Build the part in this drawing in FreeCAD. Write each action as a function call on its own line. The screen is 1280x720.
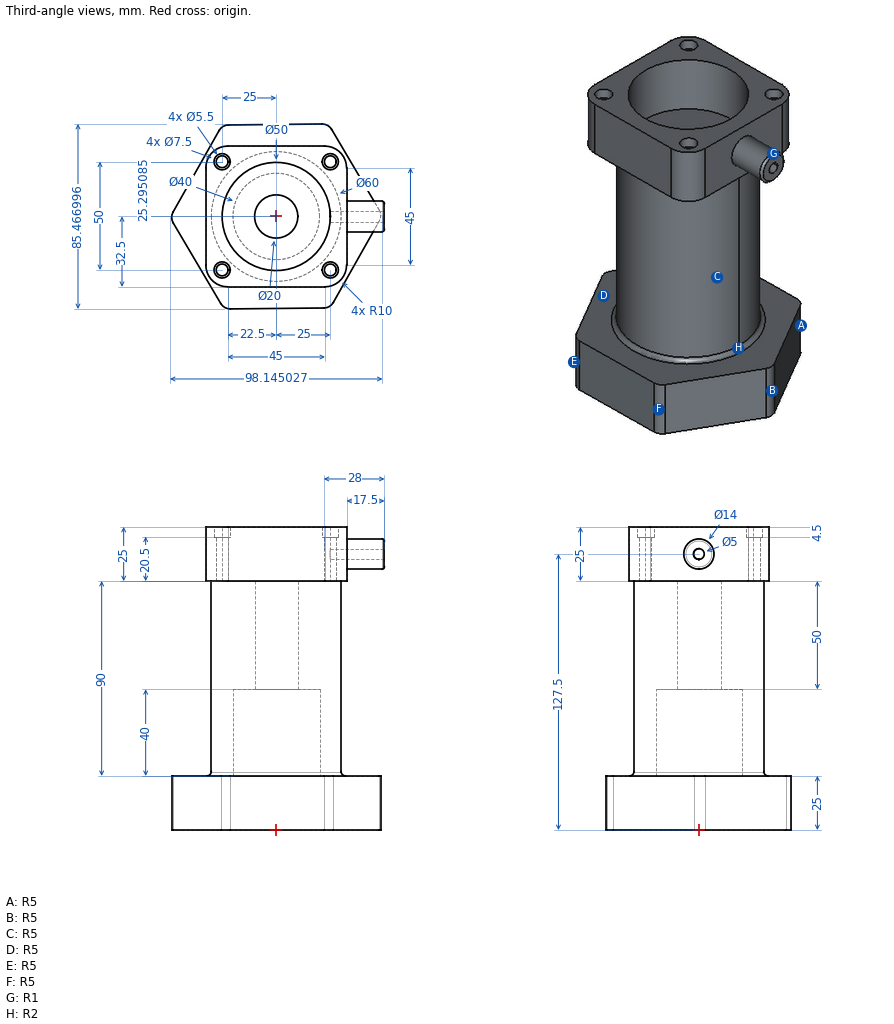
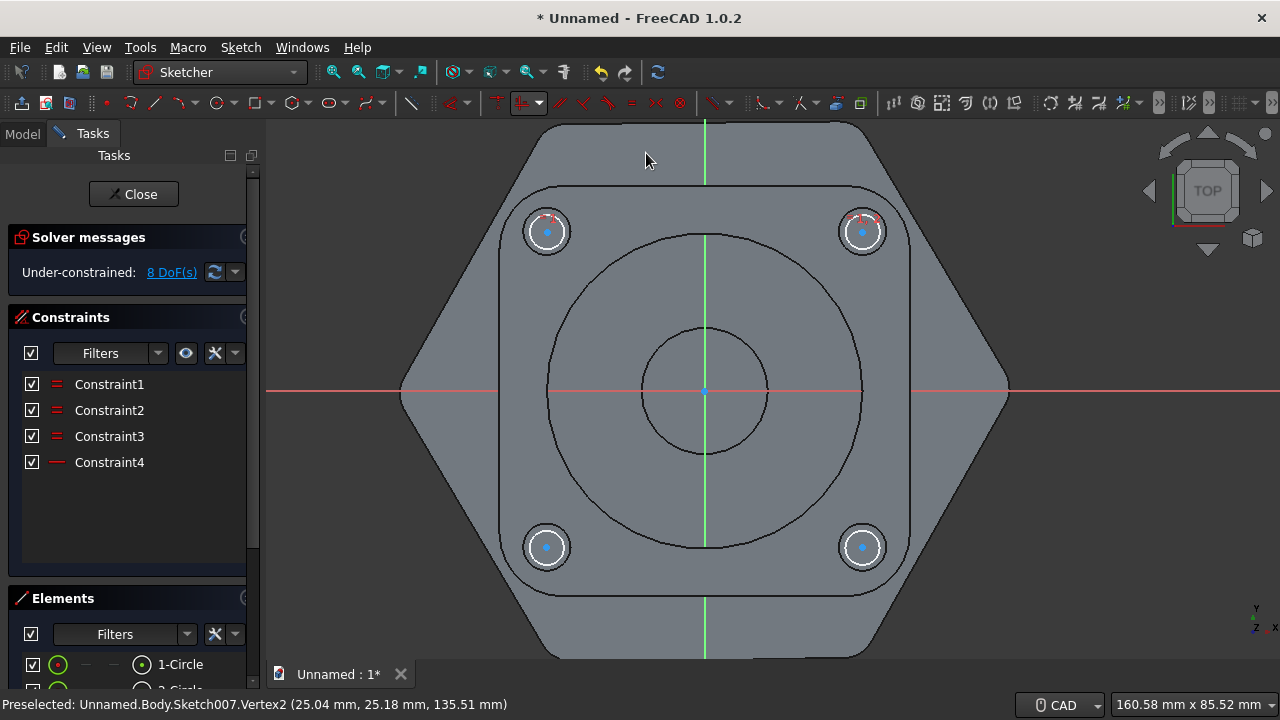
click(863, 232)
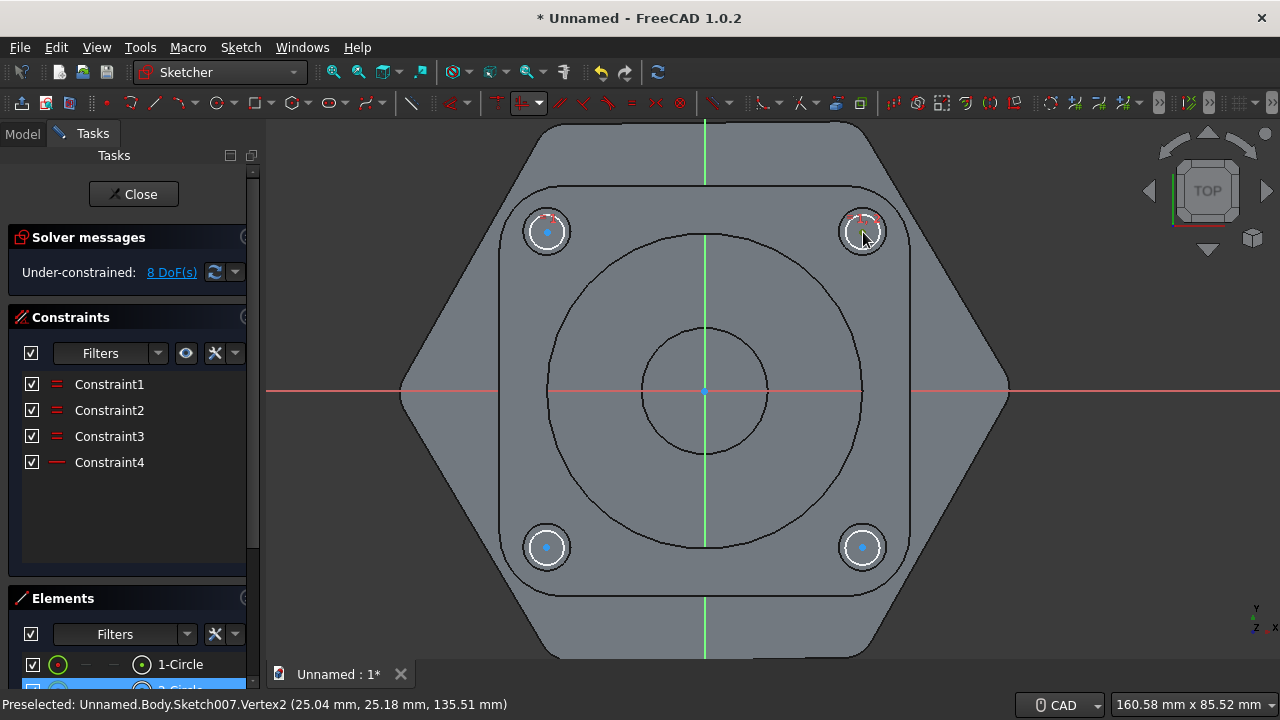
click(863, 548)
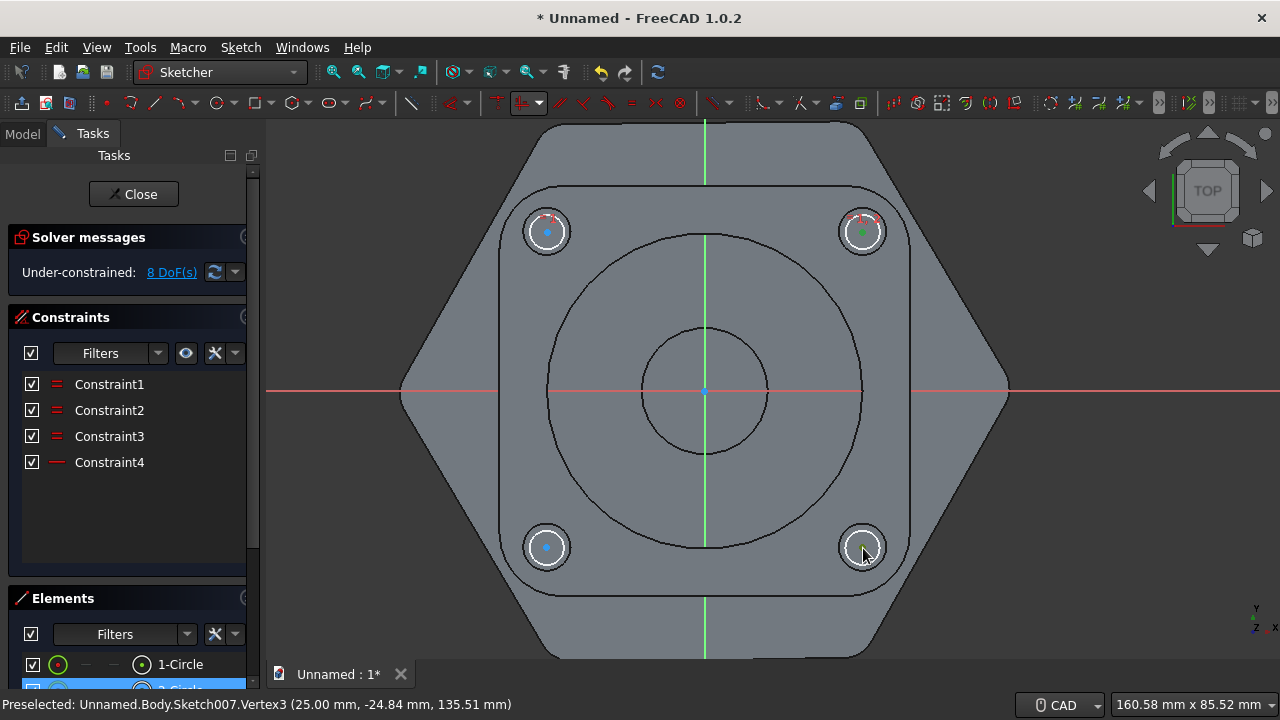
click(542, 104)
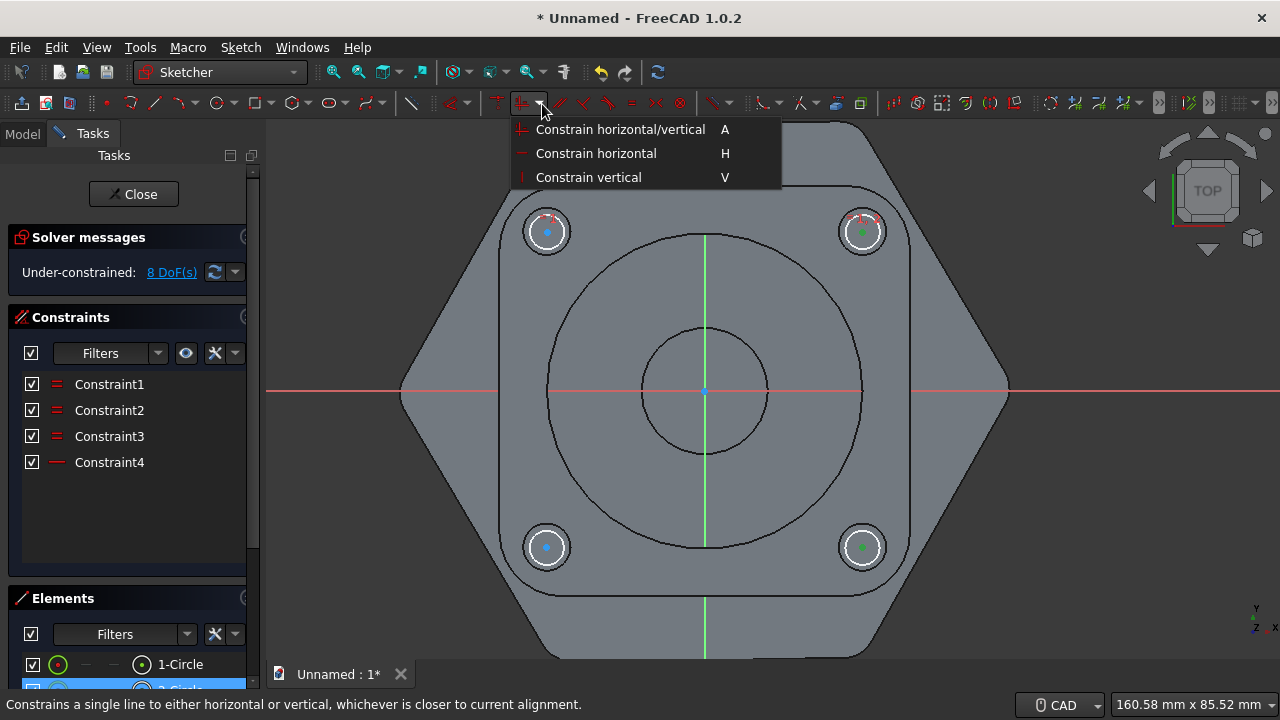
click(646, 177)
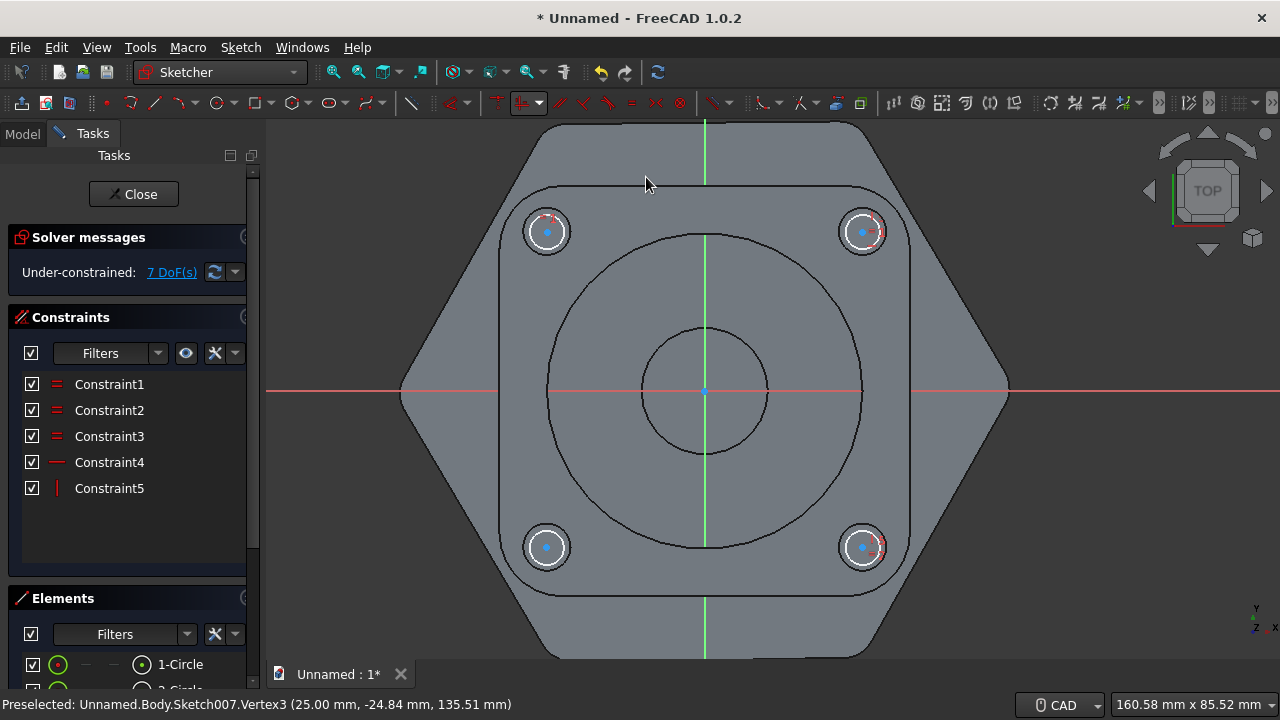
click(547, 232)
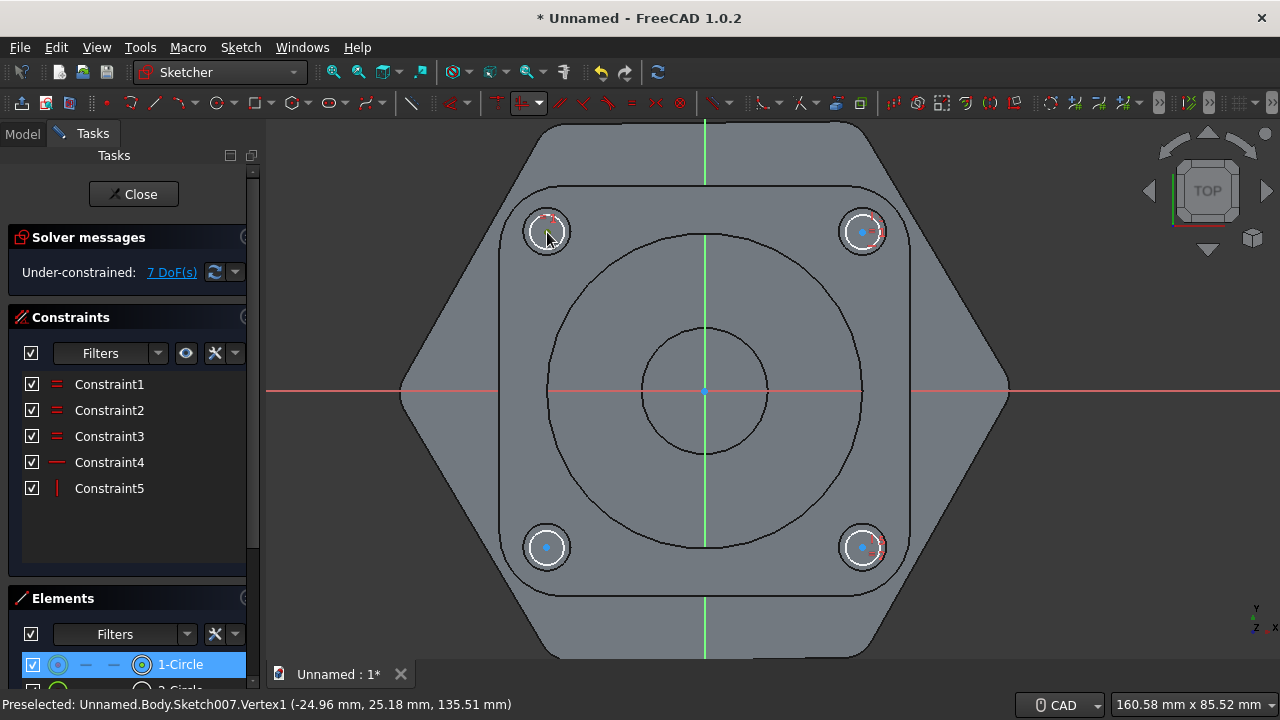
click(547, 548)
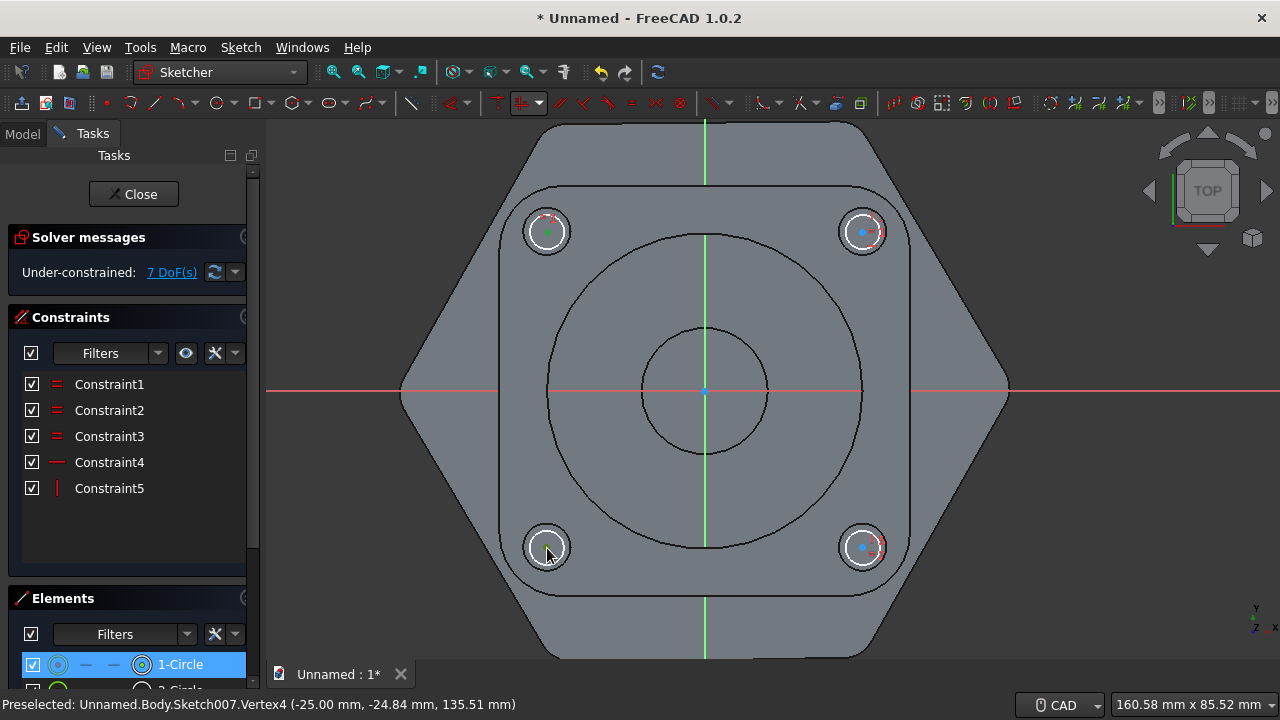
click(542, 104)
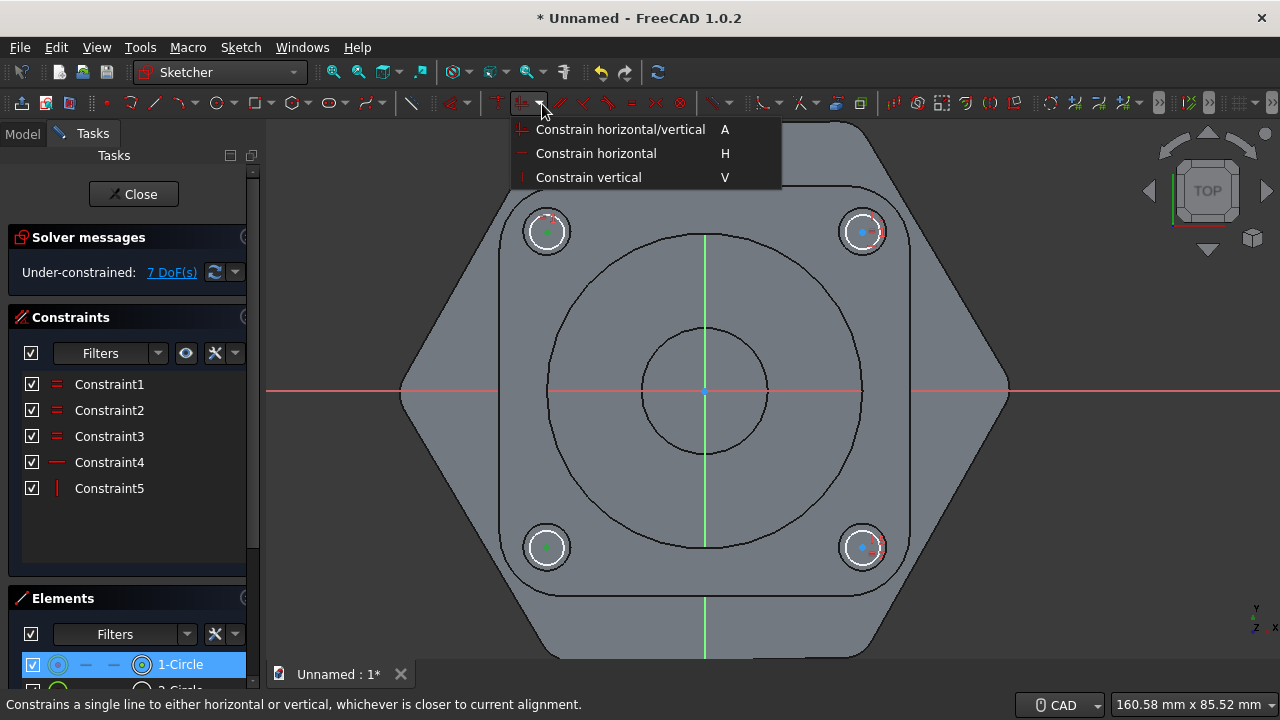
click(646, 177)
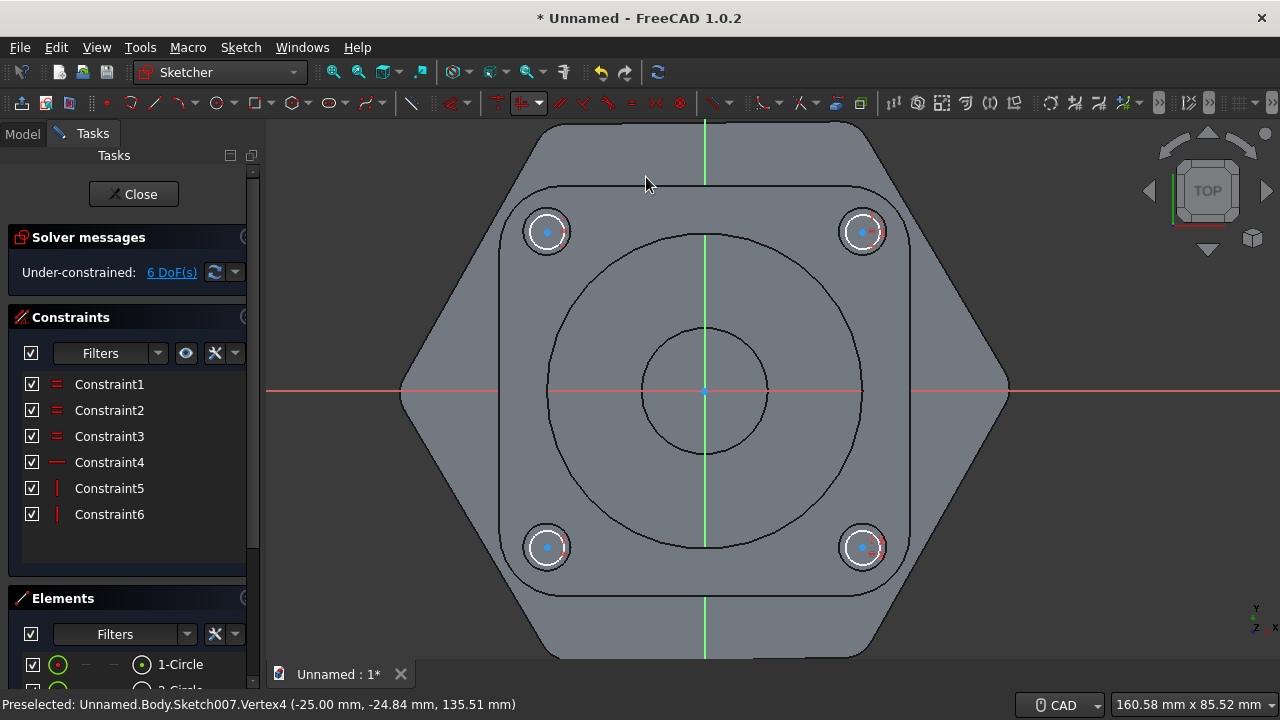
click(863, 548)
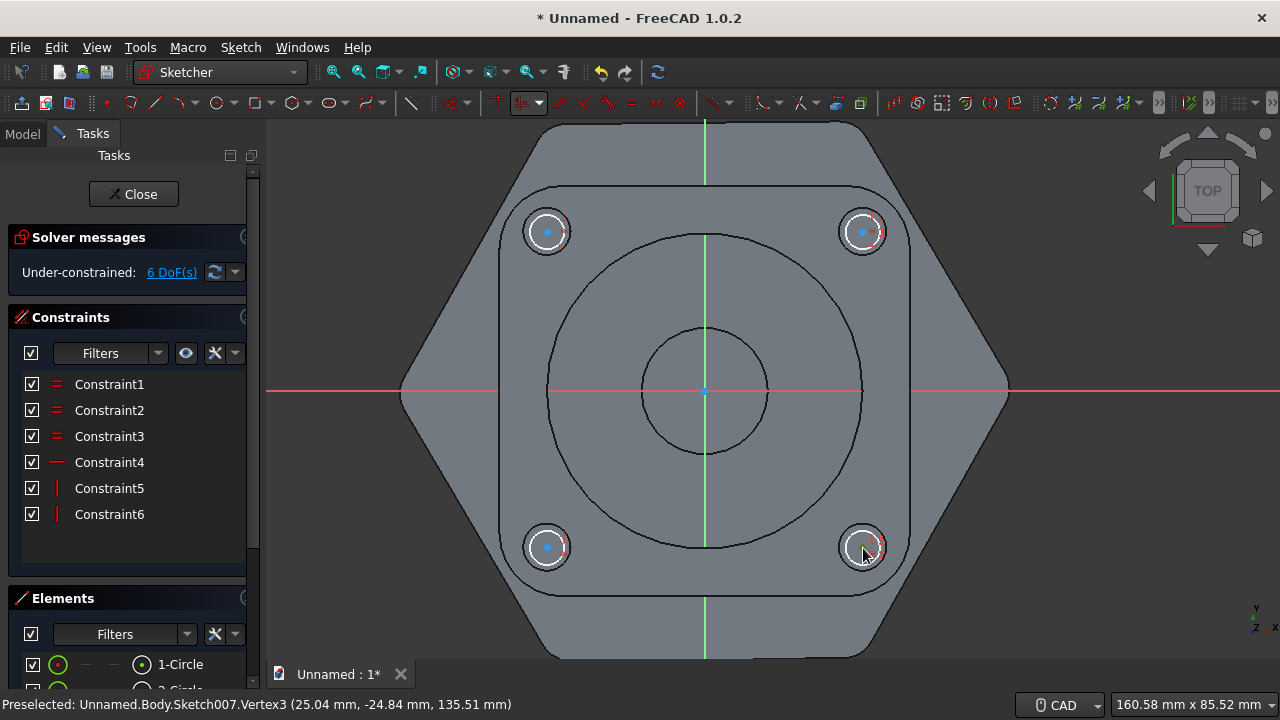
click(547, 548)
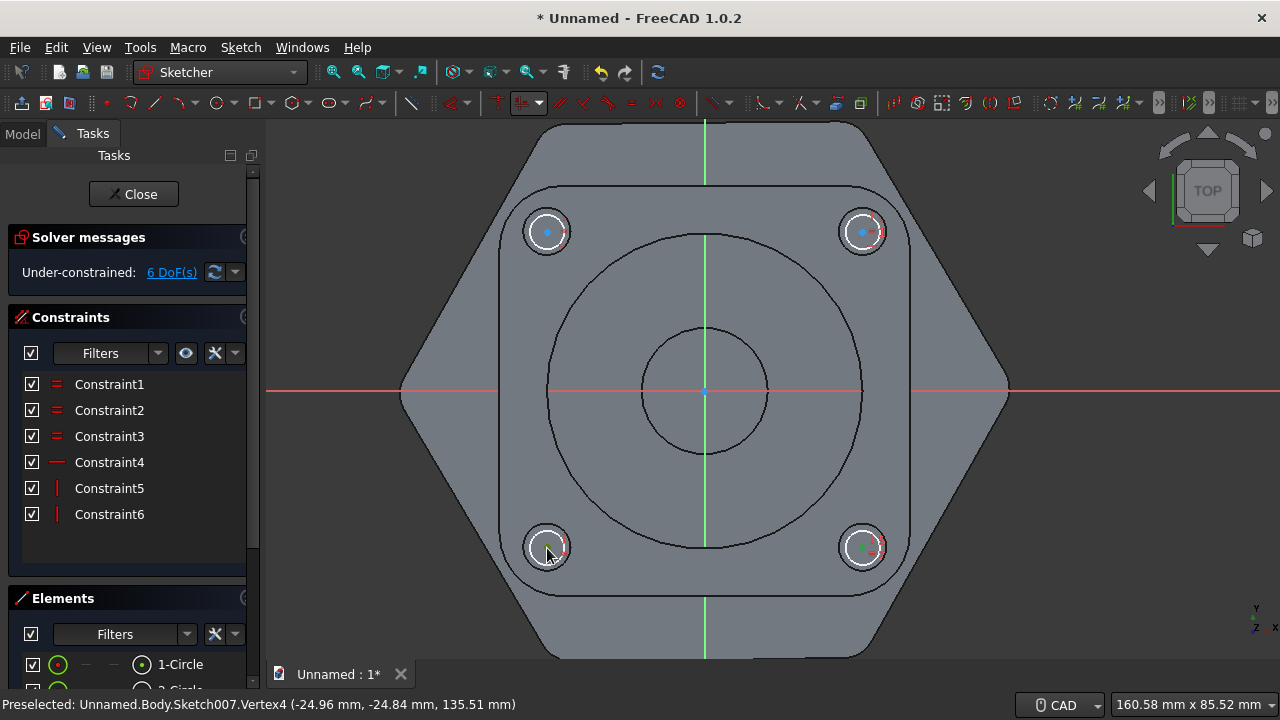
click(542, 104)